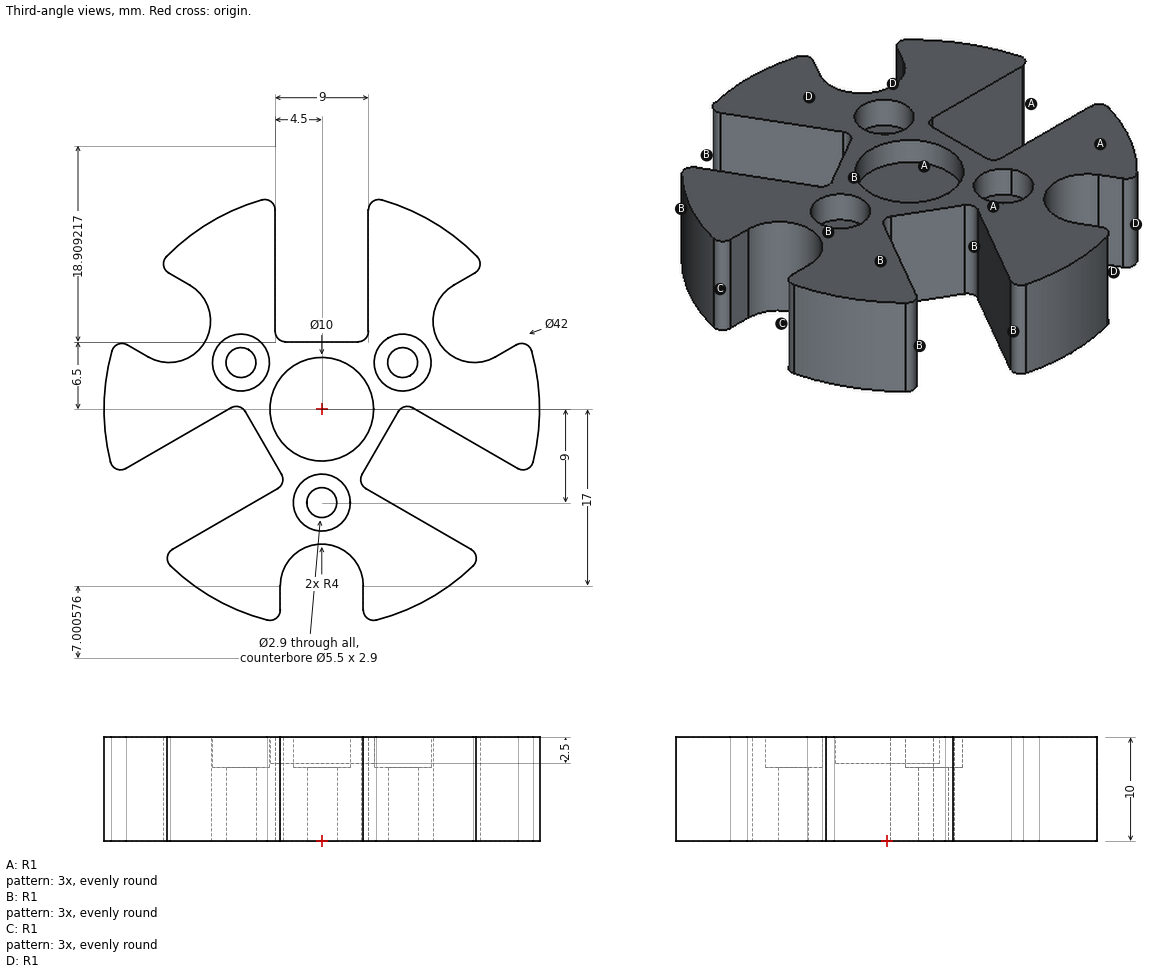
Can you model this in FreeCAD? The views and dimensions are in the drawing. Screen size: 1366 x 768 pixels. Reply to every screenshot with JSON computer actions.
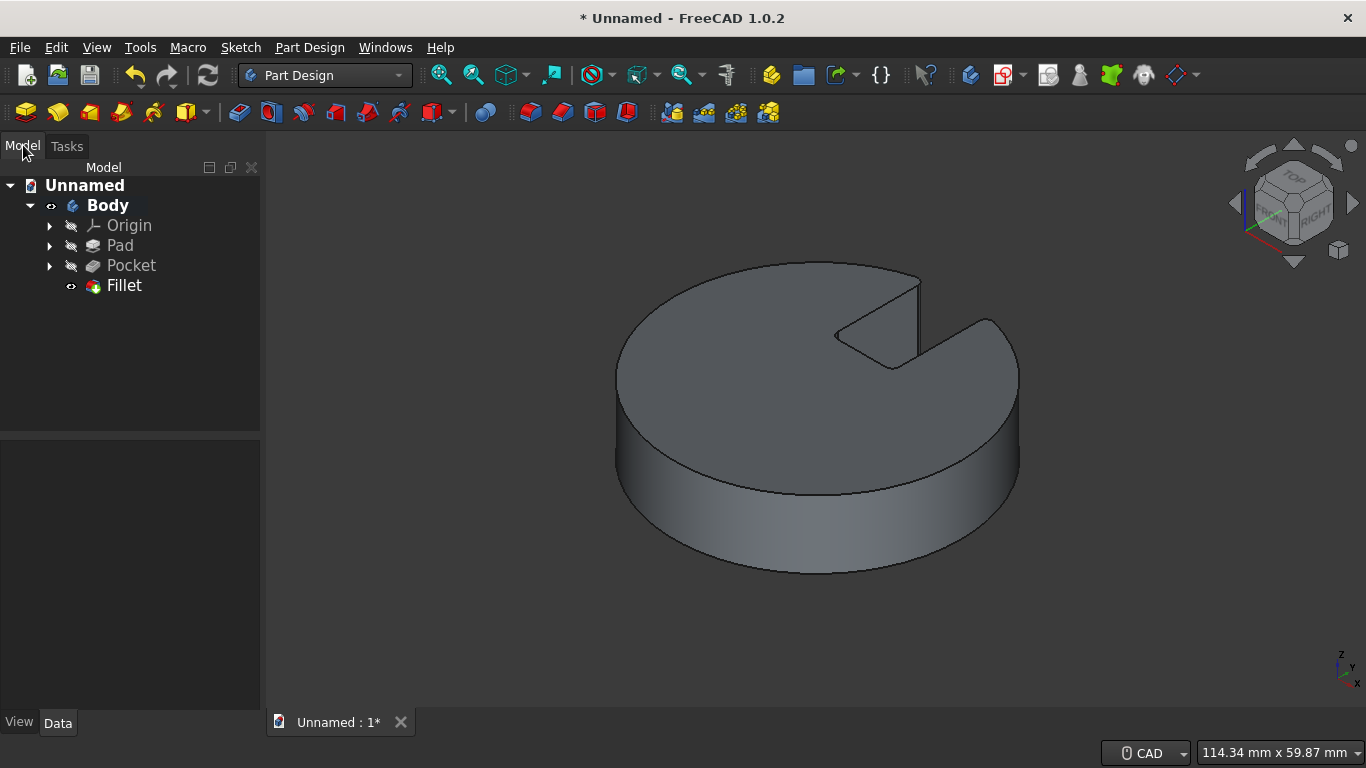
{"action": "left_click", "coordinate": [116, 266]}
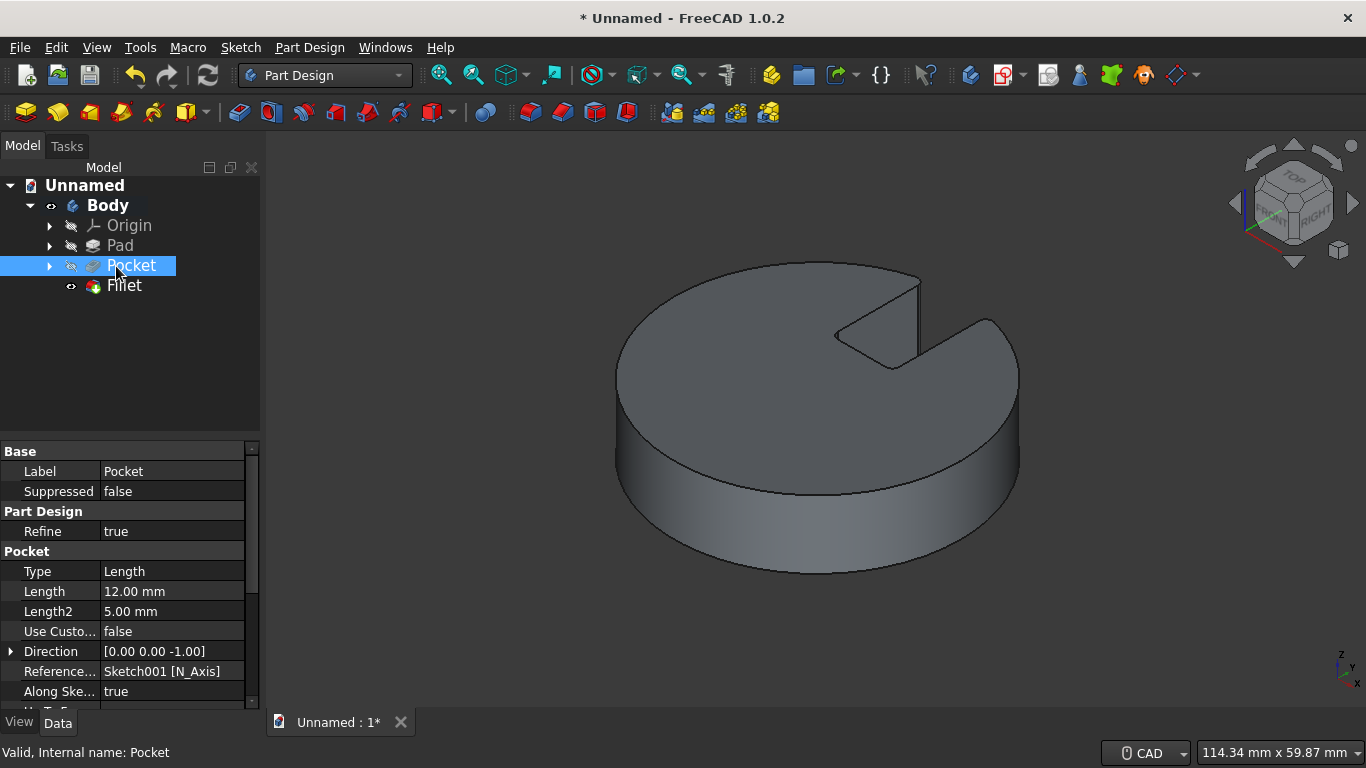
{"action": "left_click", "coordinate": [736, 112]}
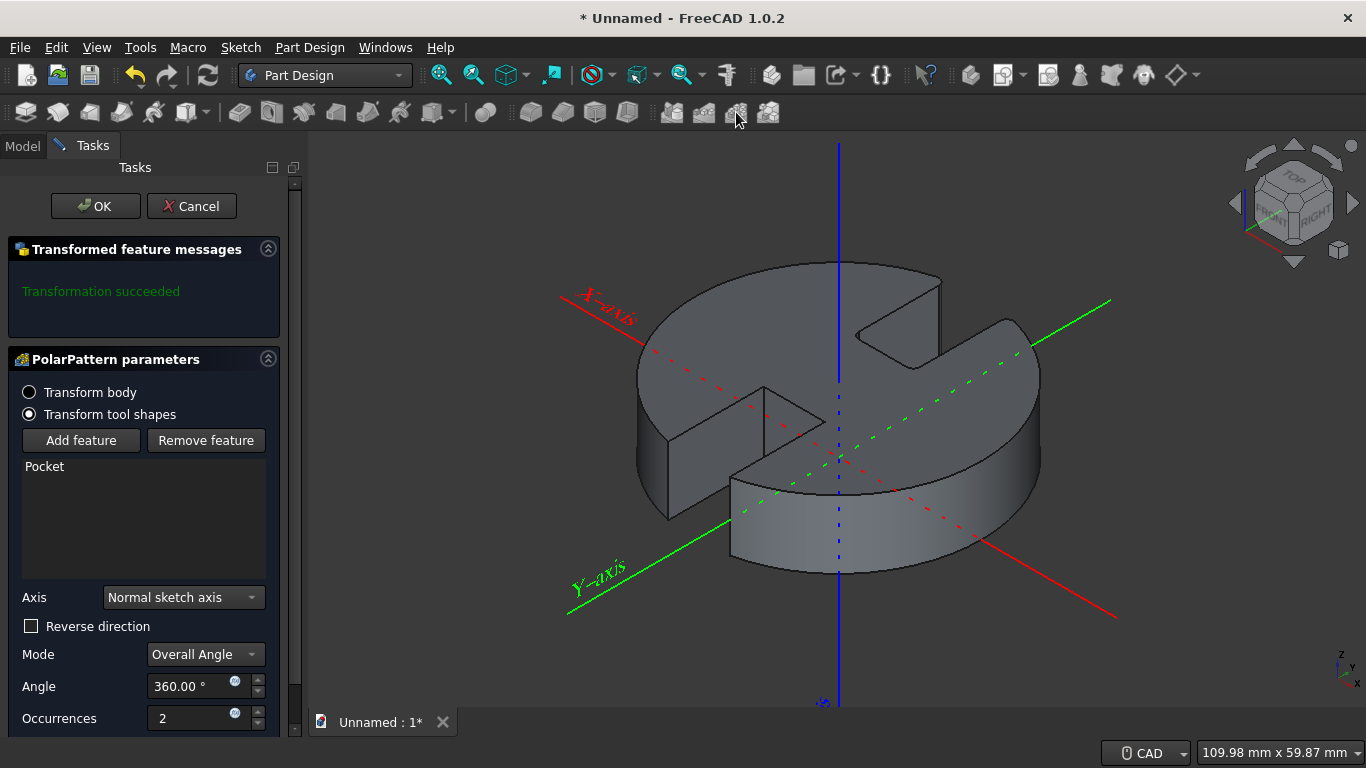
{"action": "left_click", "coordinate": [184, 598]}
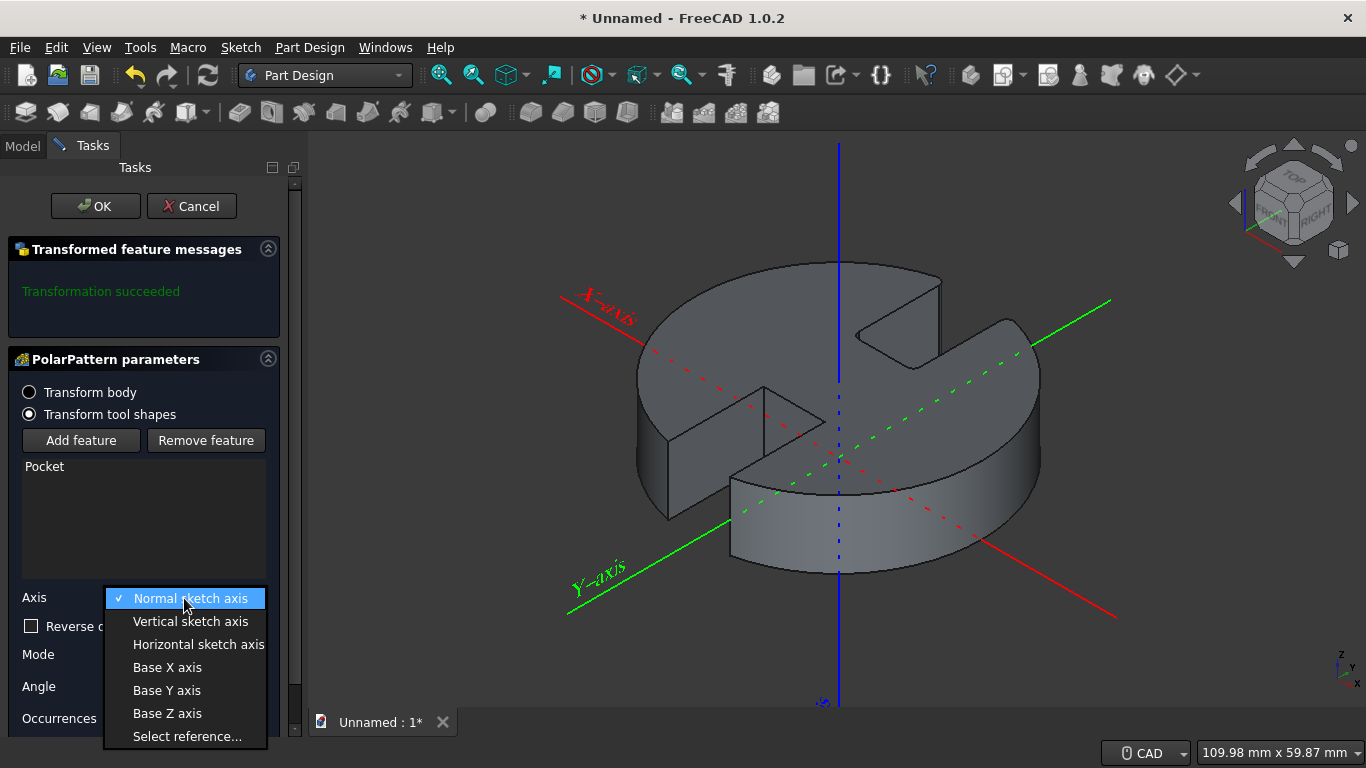
{"action": "left_click", "coordinate": [184, 714]}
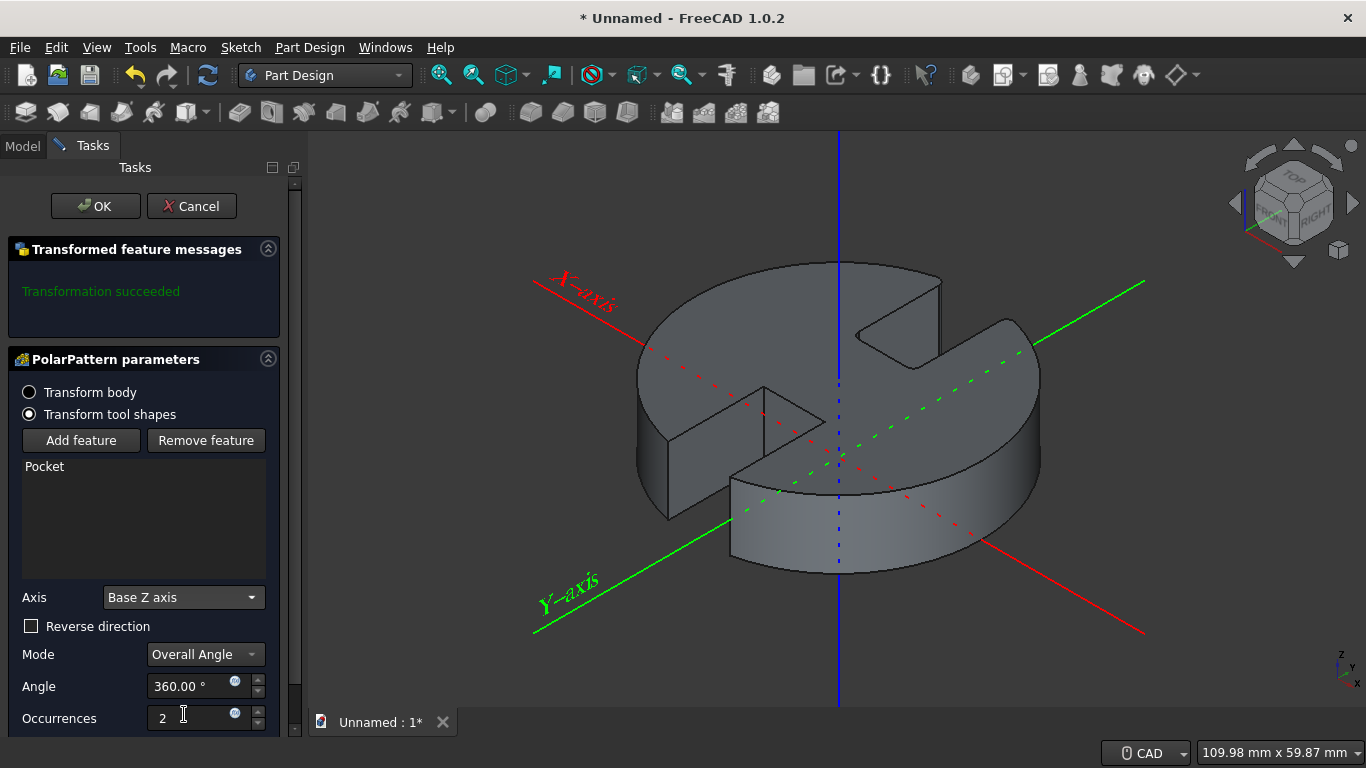
{"action": "triple_click", "coordinate": [198, 718]}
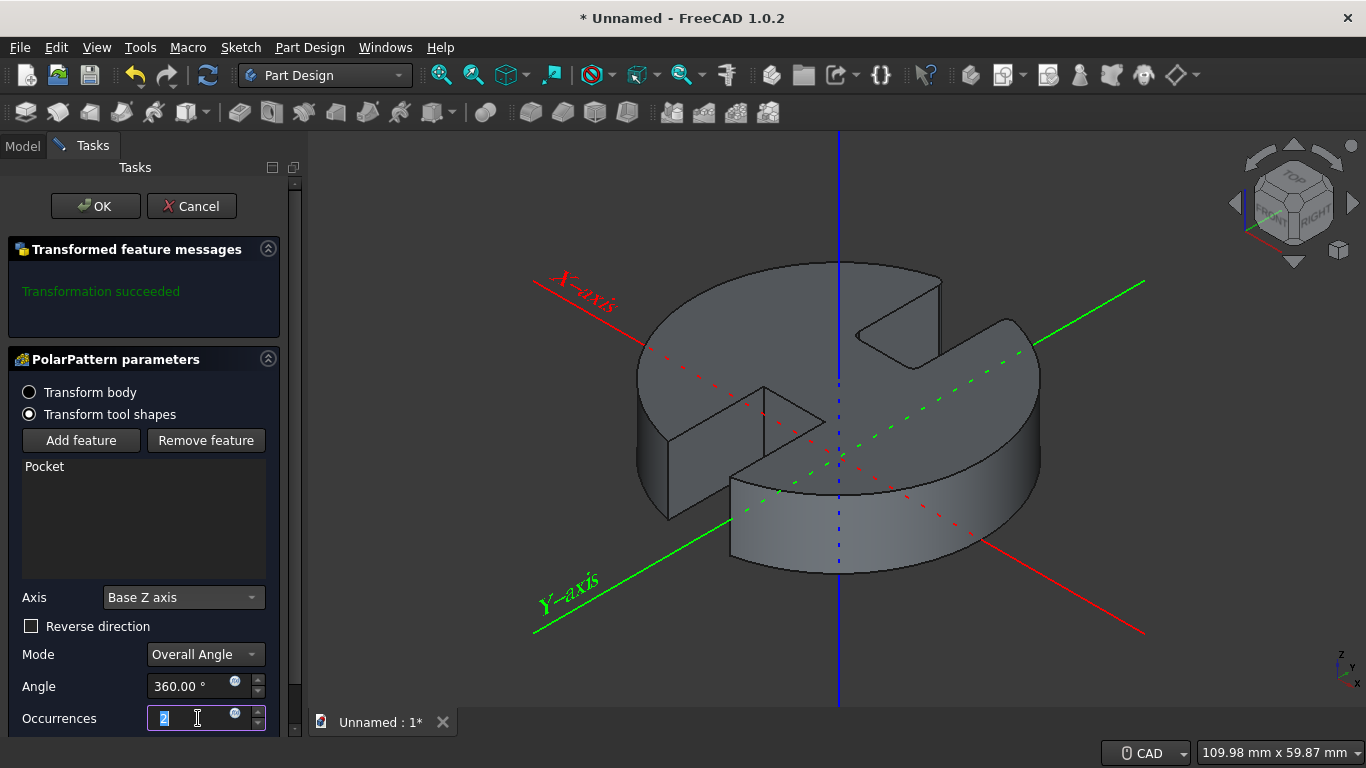
{"action": "type", "text": "3"}
{"action": "key", "text": "Tab"}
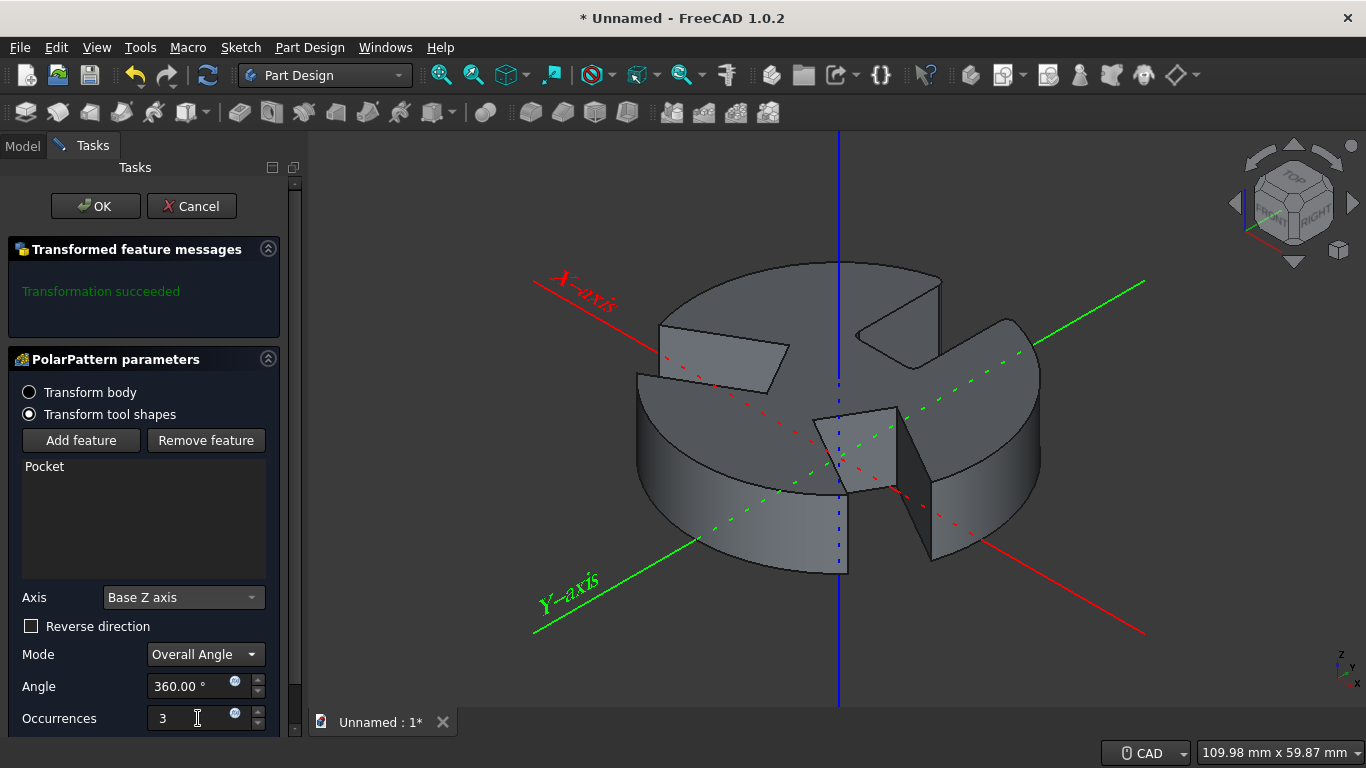
{"action": "left_click", "coordinate": [96, 206]}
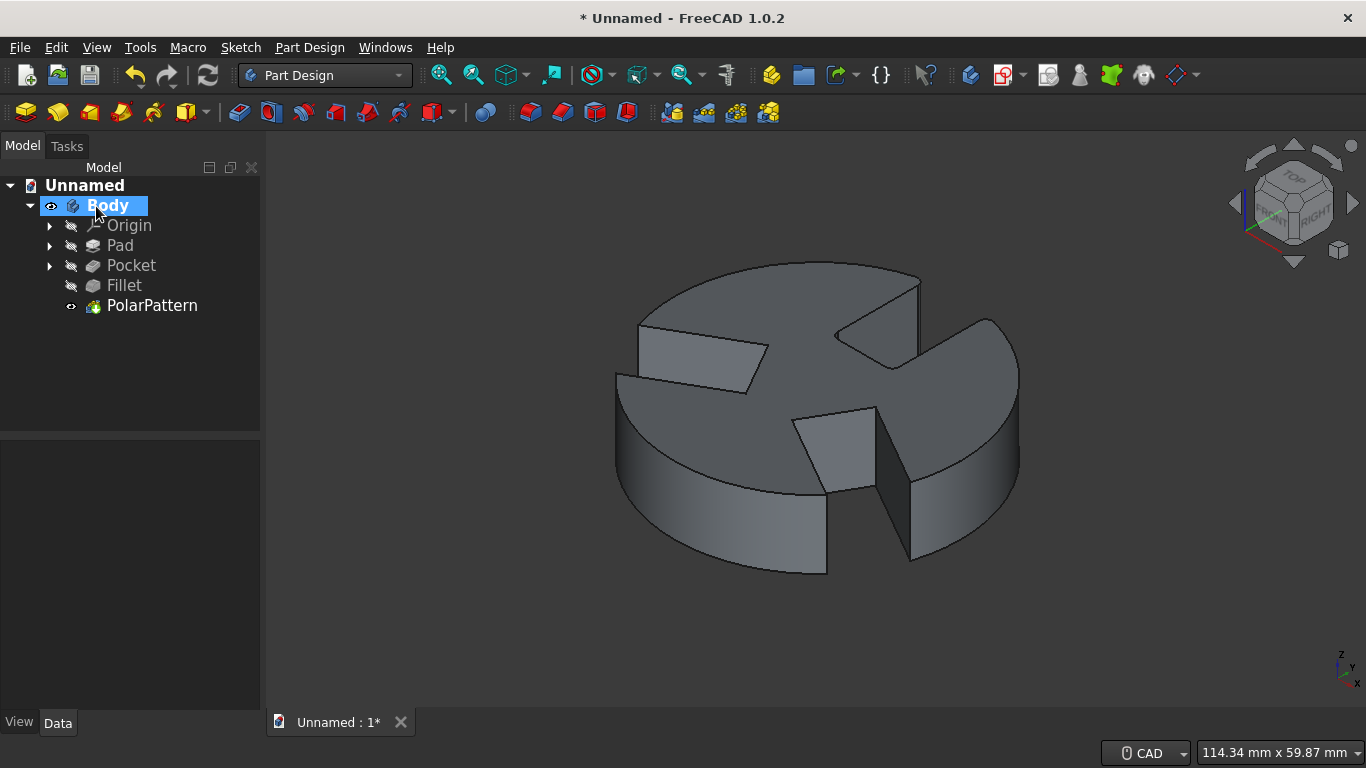
{"action": "left_click", "coordinate": [910, 521]}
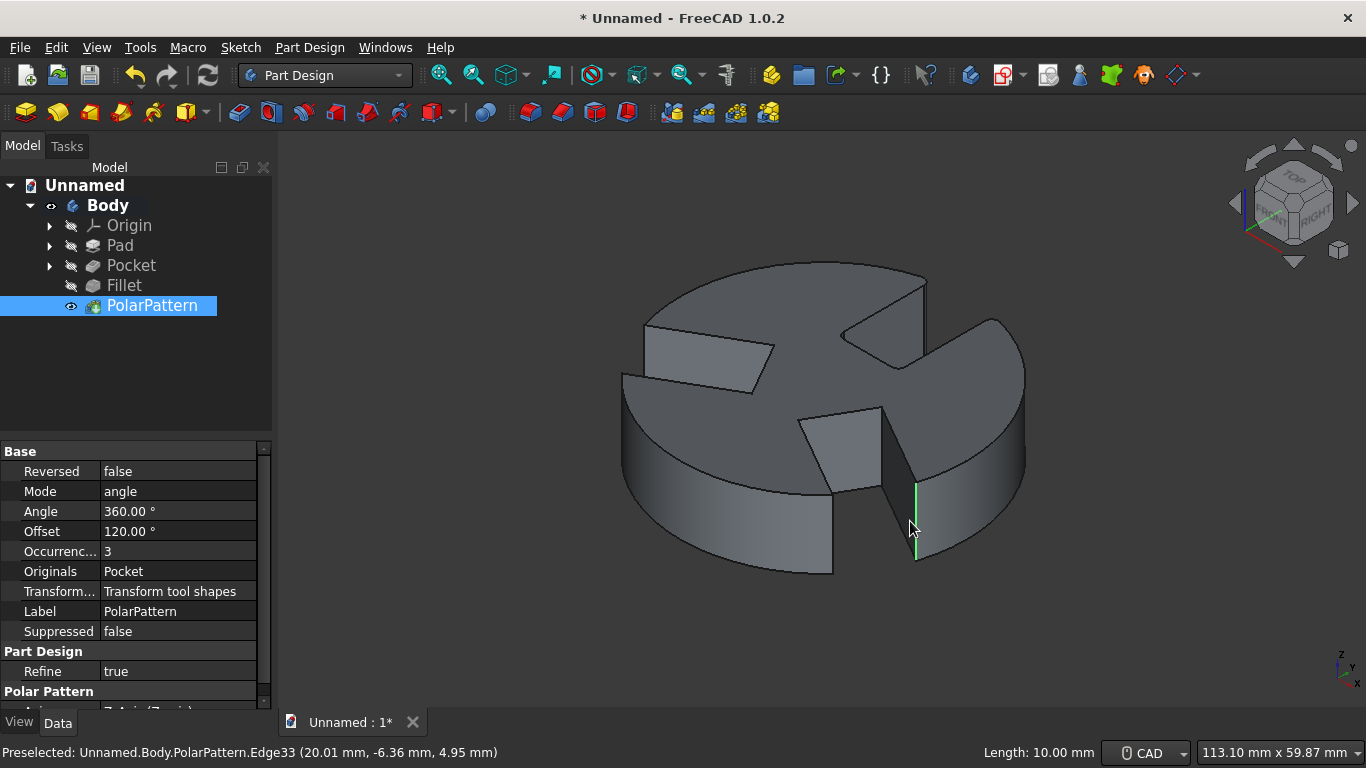
{"action": "left_click", "coordinate": [833, 534], "text": "ctrl"}